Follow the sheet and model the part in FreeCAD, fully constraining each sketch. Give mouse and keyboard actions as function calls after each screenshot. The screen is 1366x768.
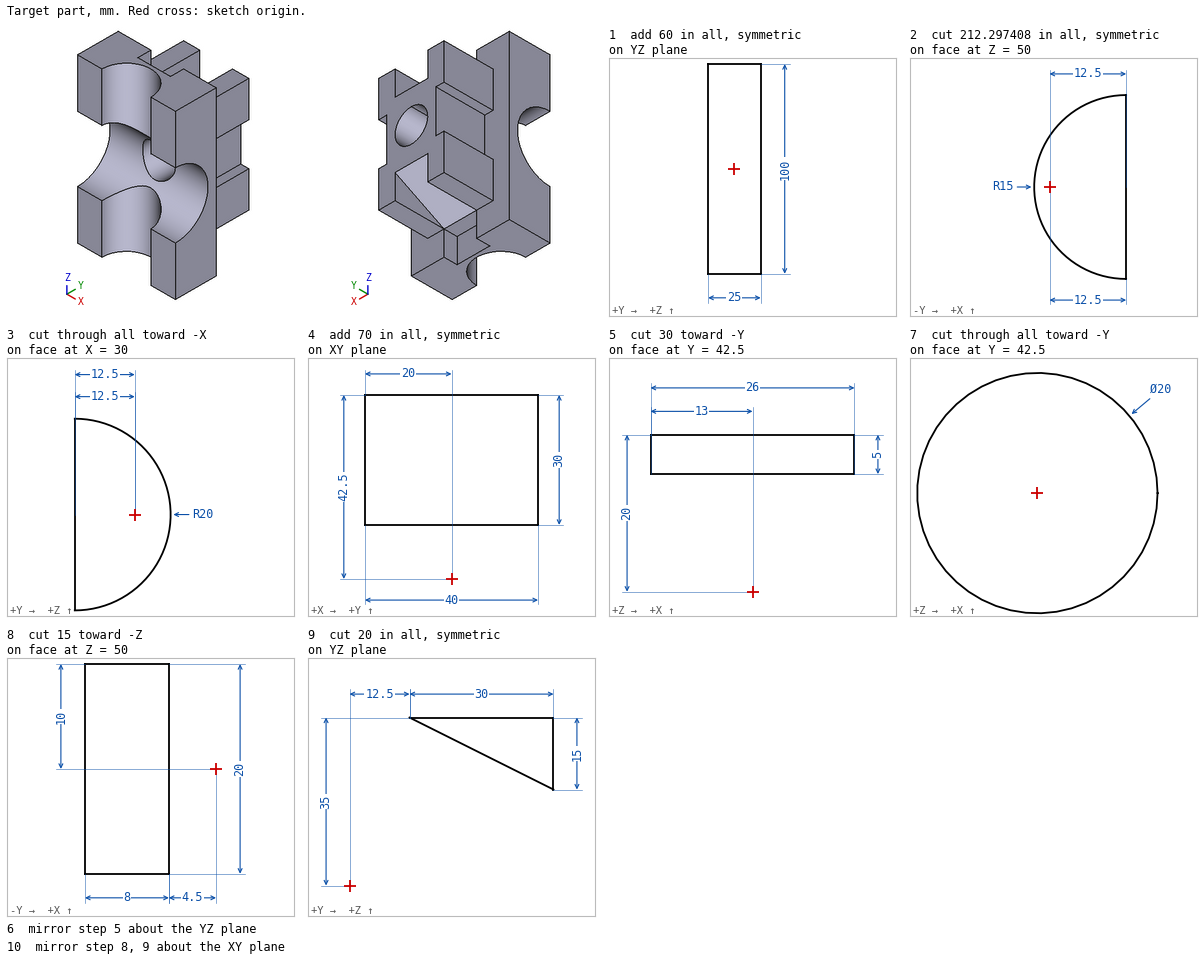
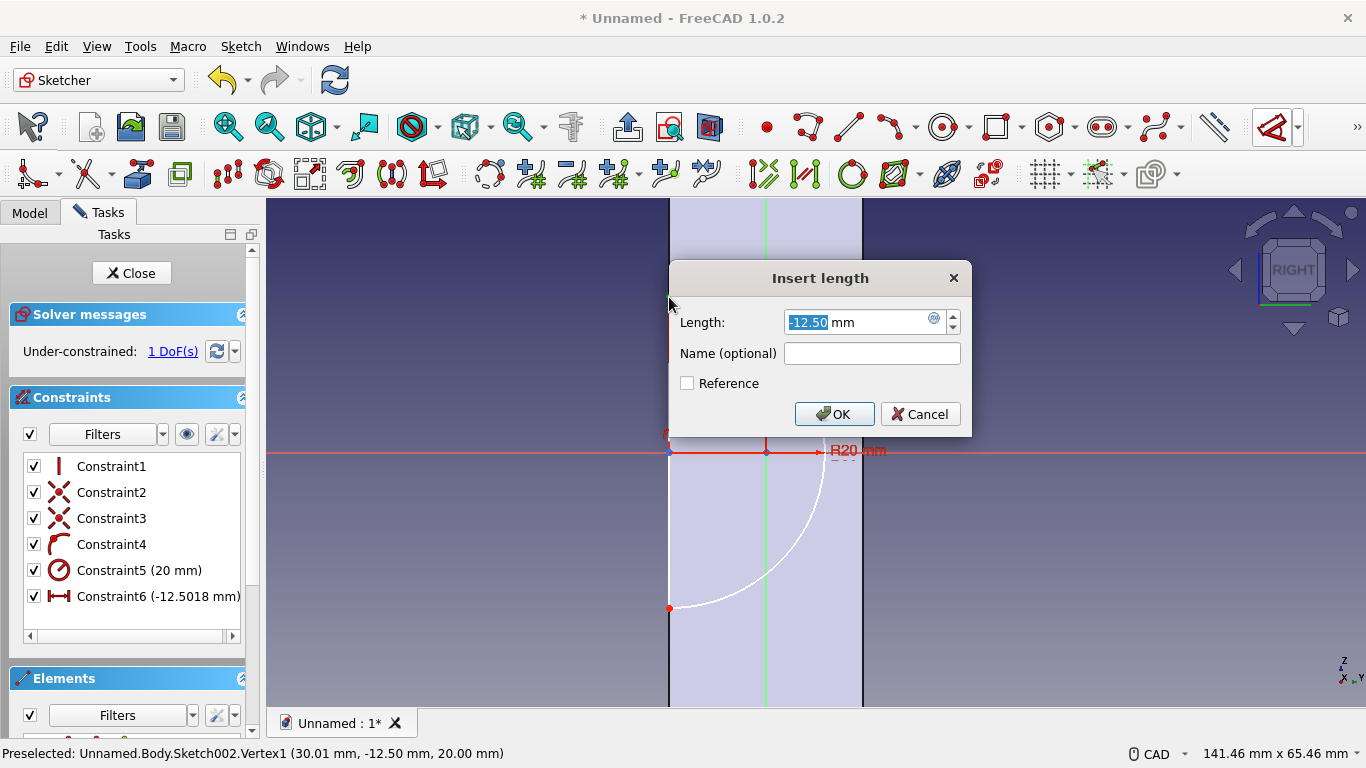
text(-12.5)
key(Return)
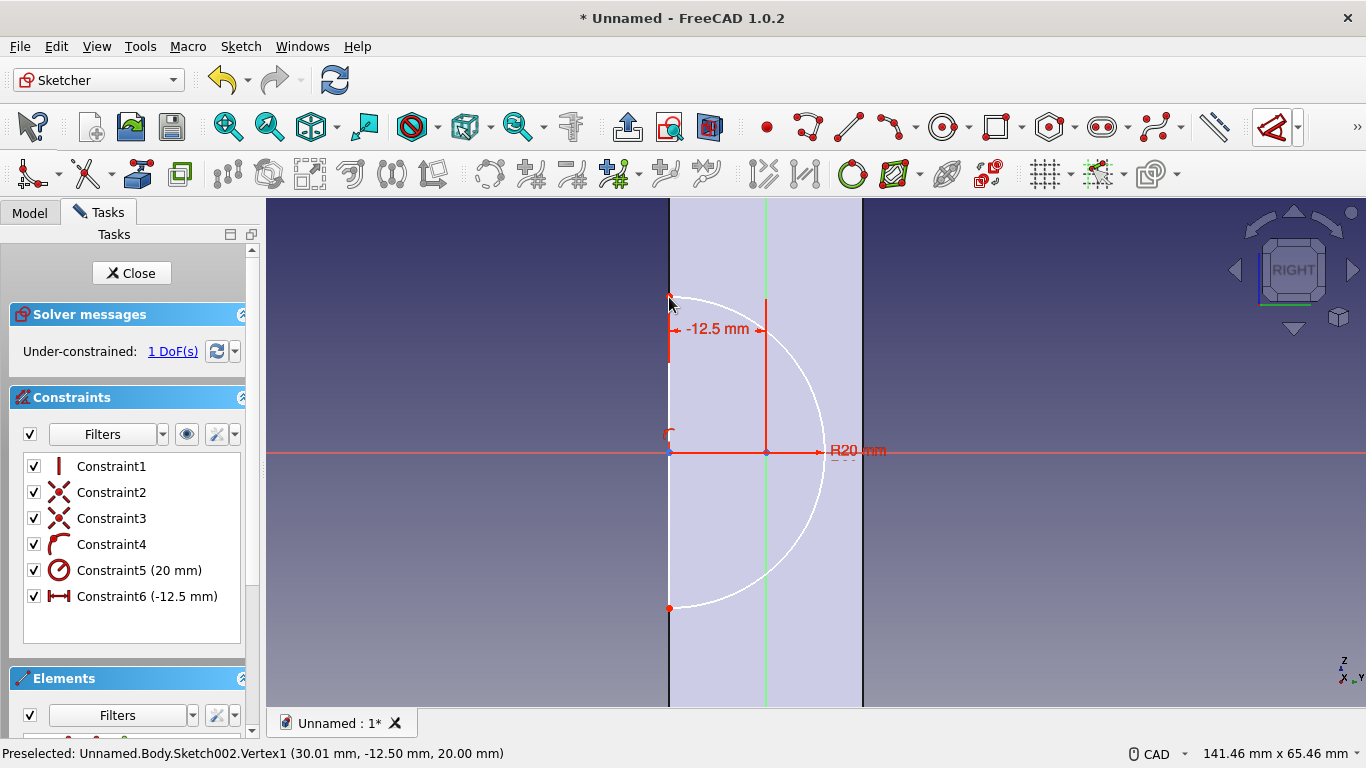
click(669, 452)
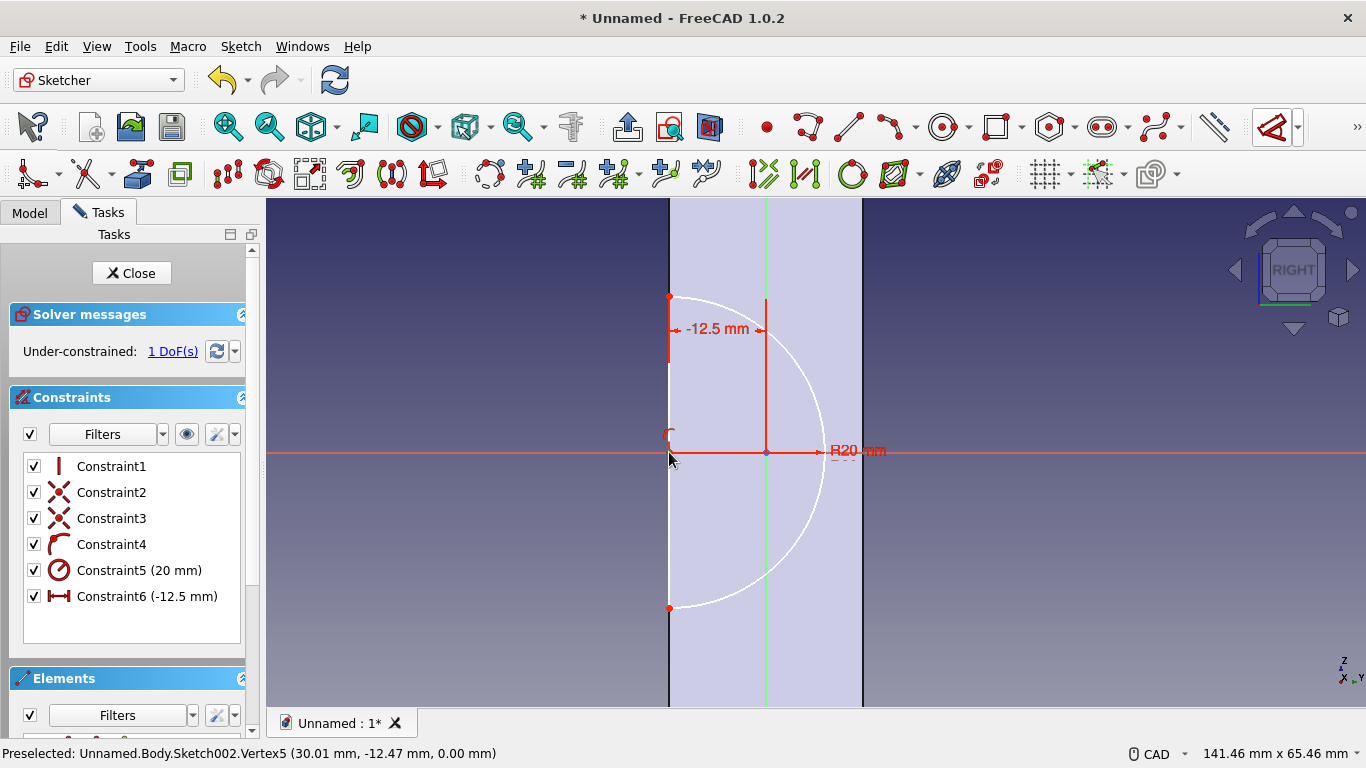
key(l)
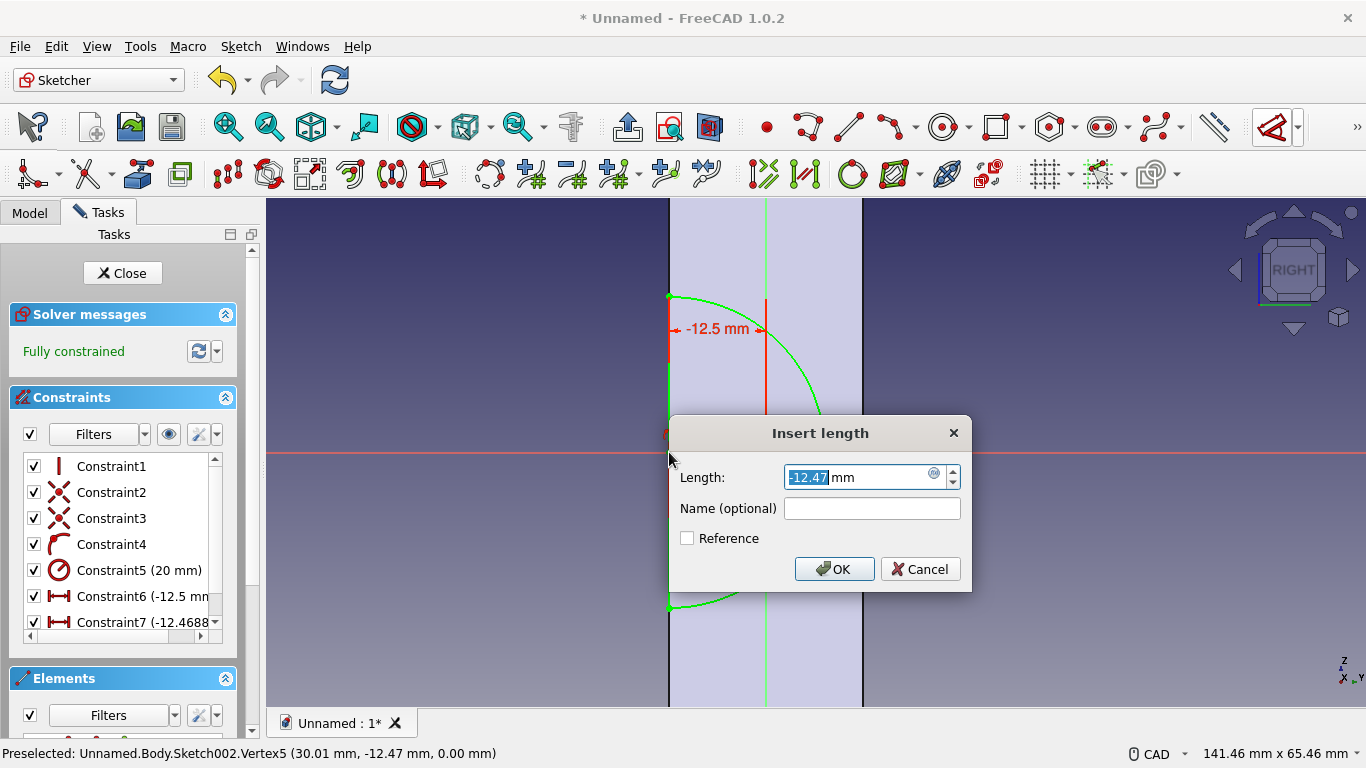
text(-12.5)
key(Return)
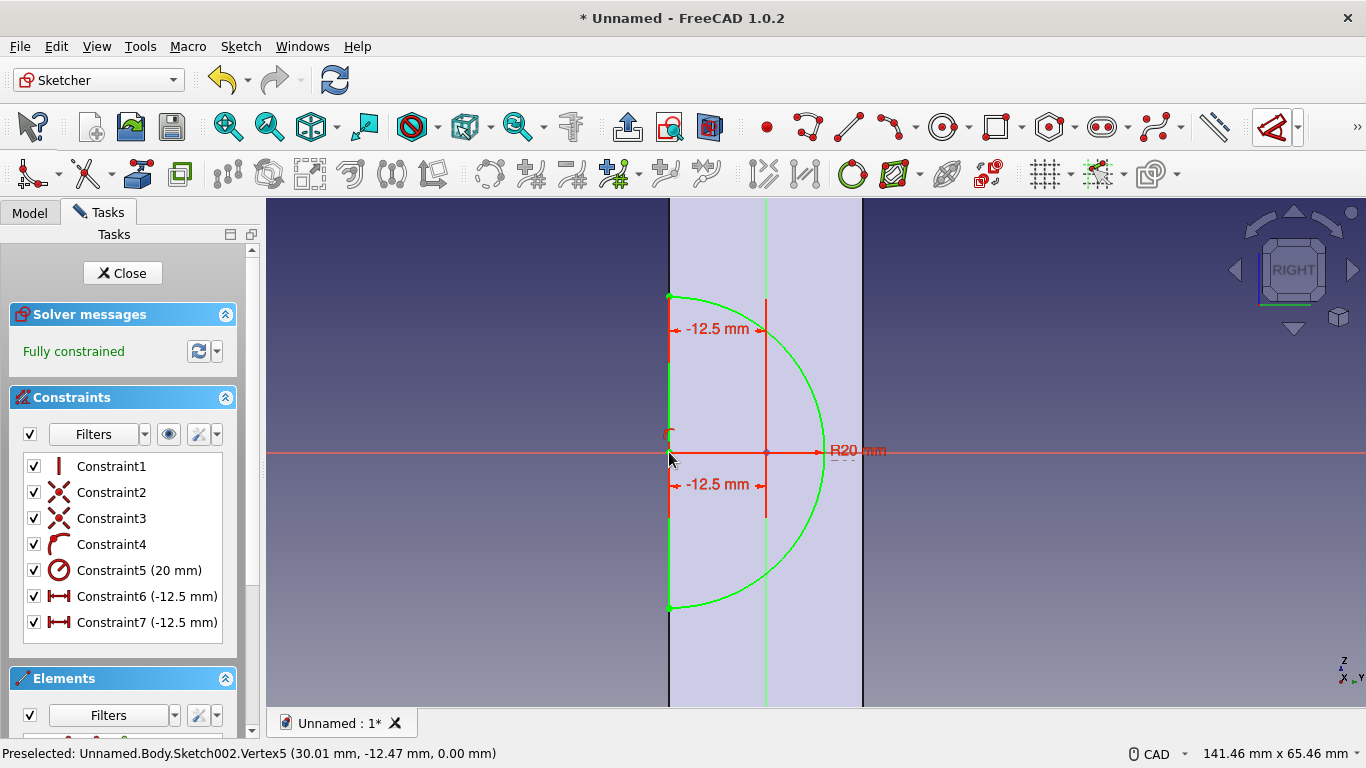
click(123, 273)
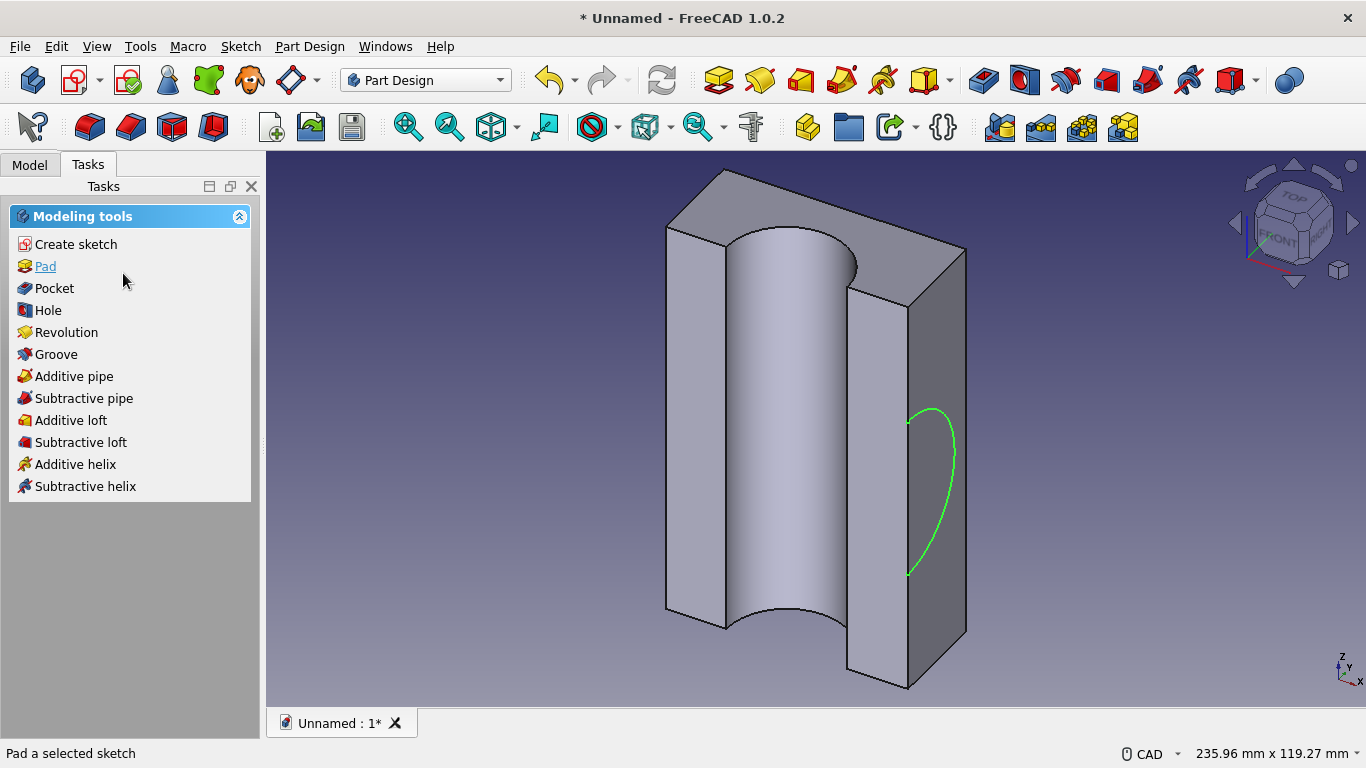
click(984, 80)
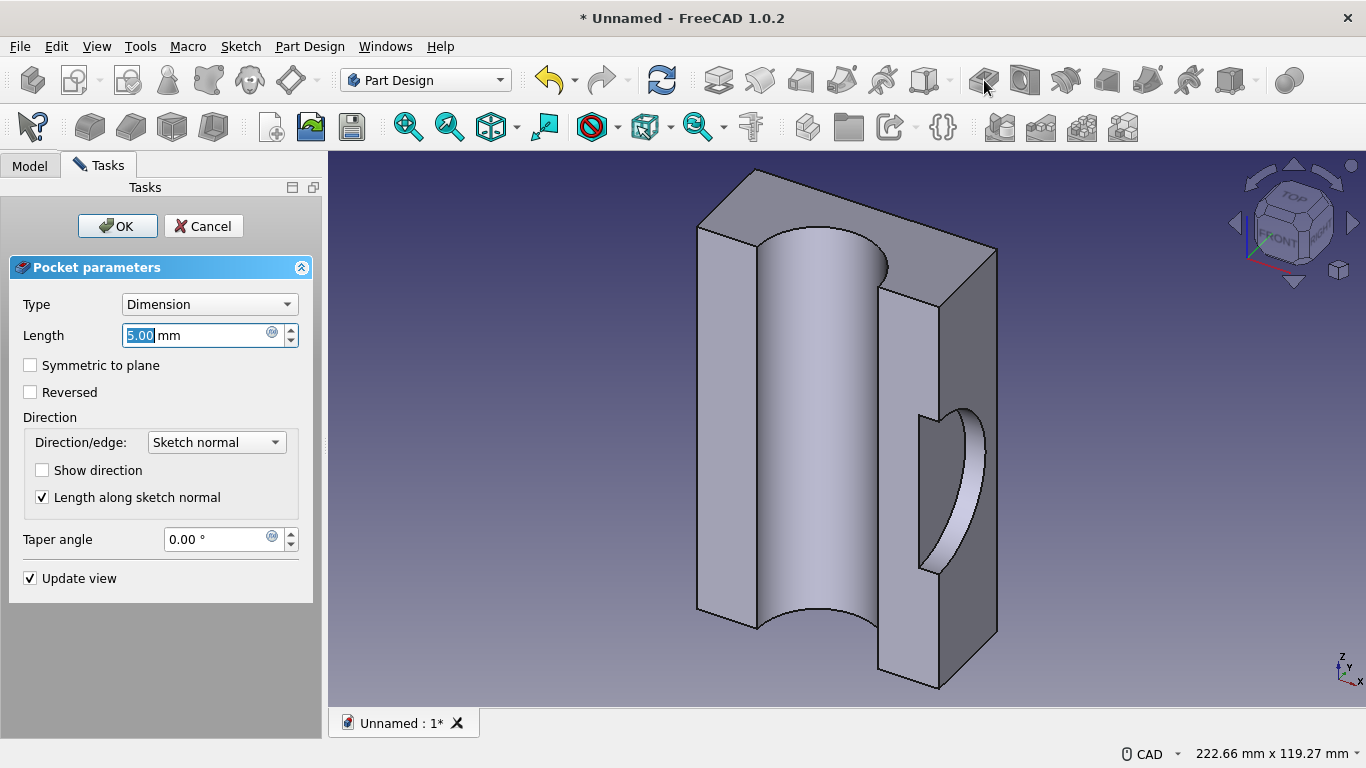
click(210, 304)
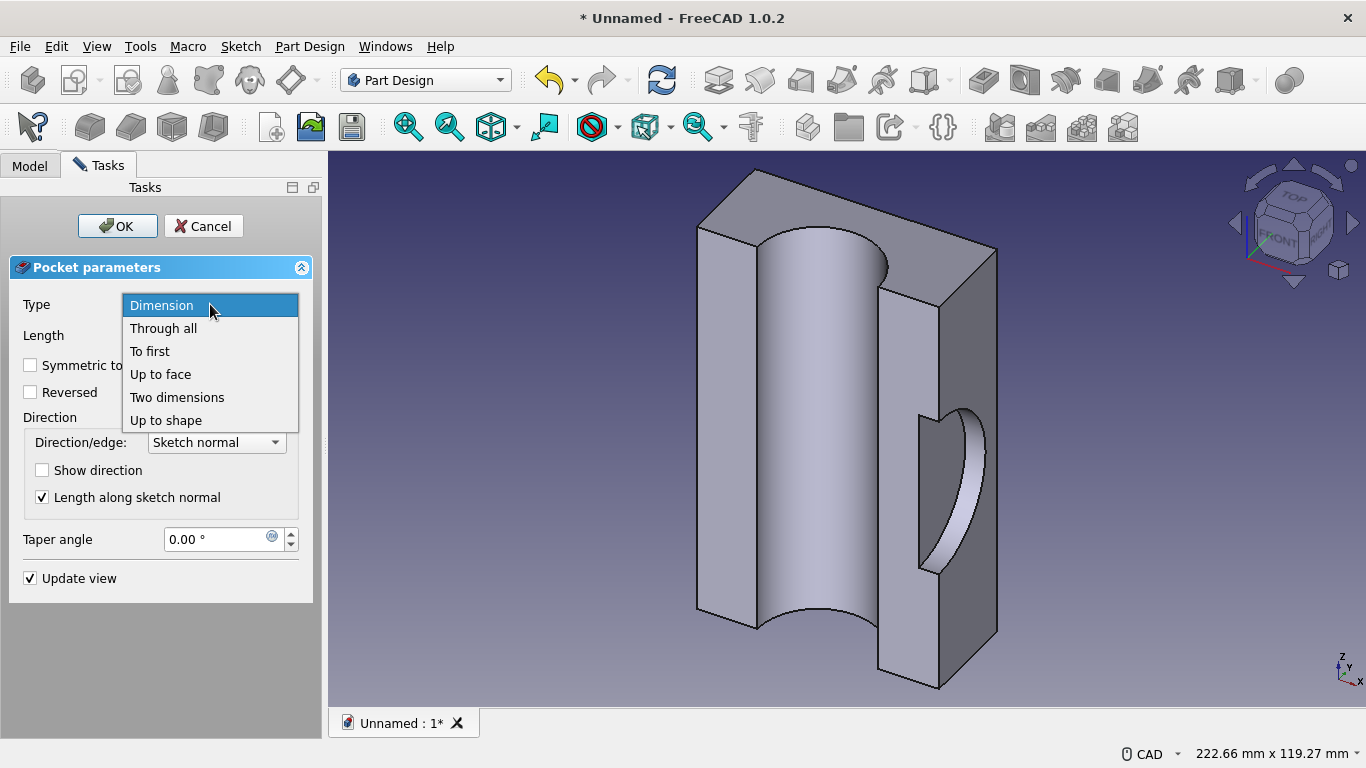
click(208, 328)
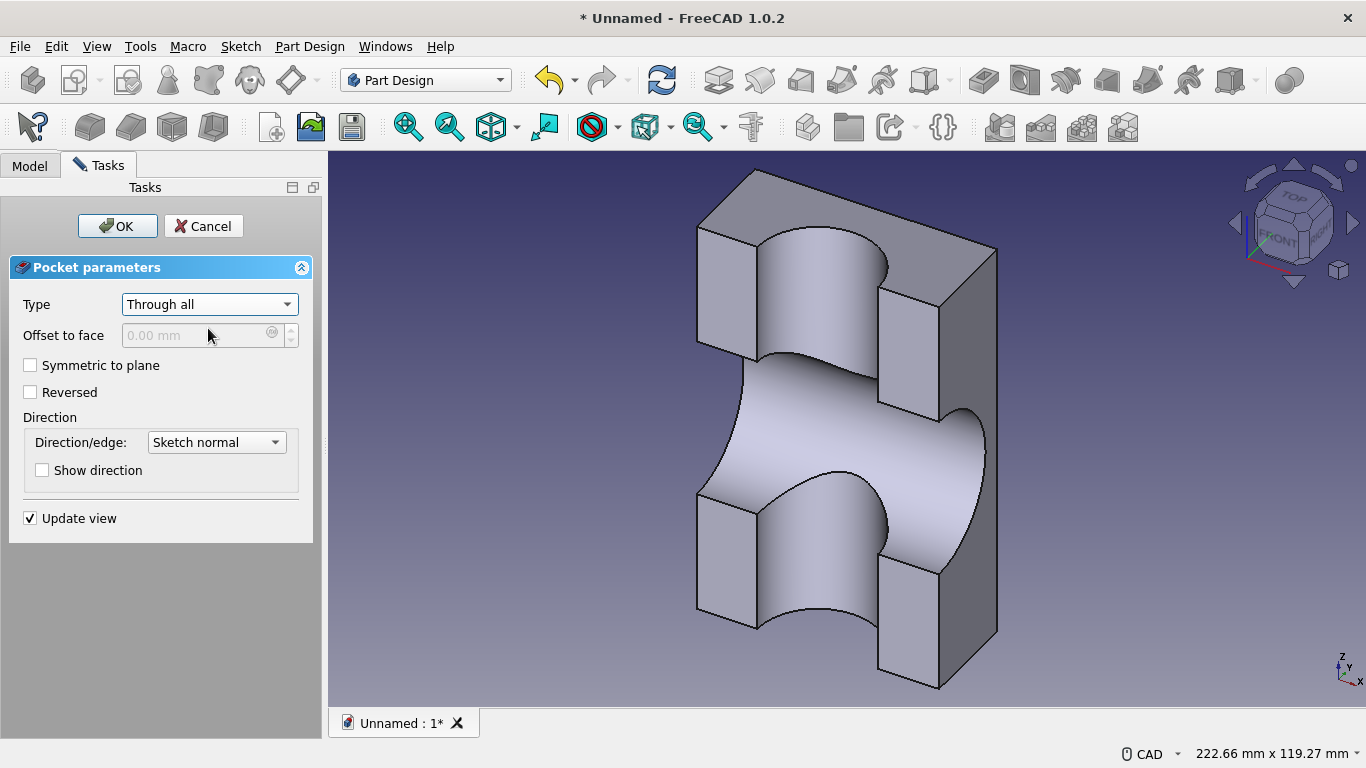
click(118, 226)